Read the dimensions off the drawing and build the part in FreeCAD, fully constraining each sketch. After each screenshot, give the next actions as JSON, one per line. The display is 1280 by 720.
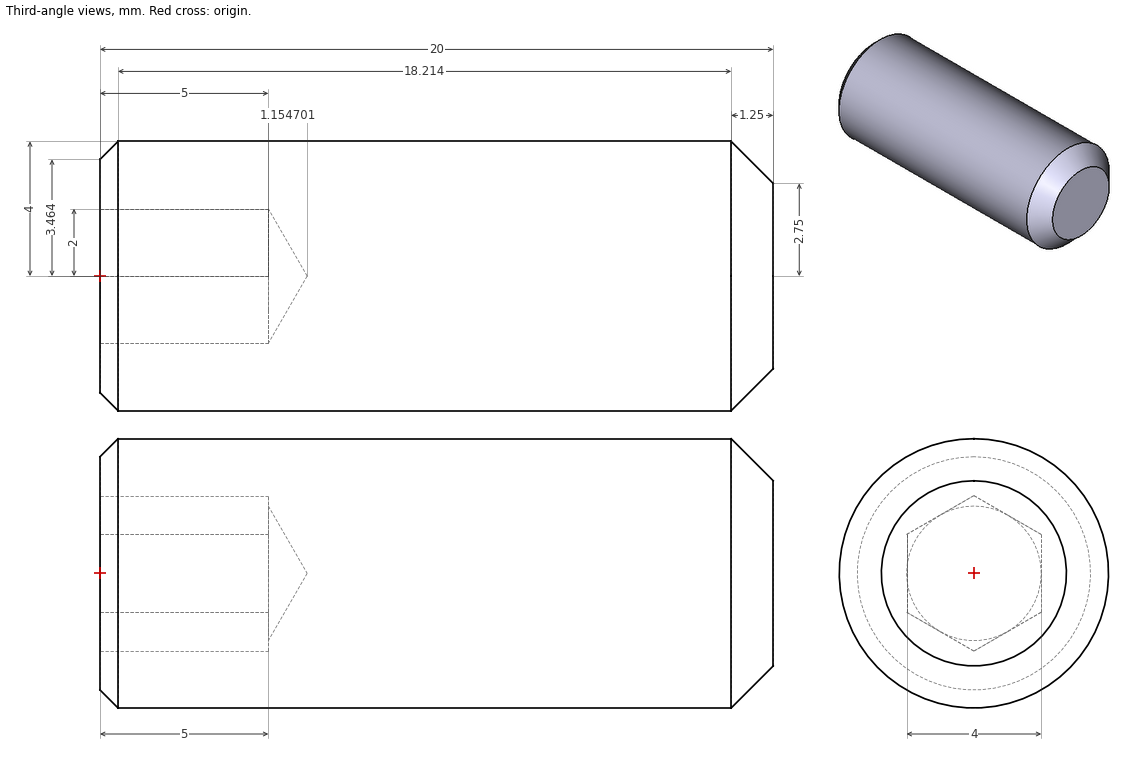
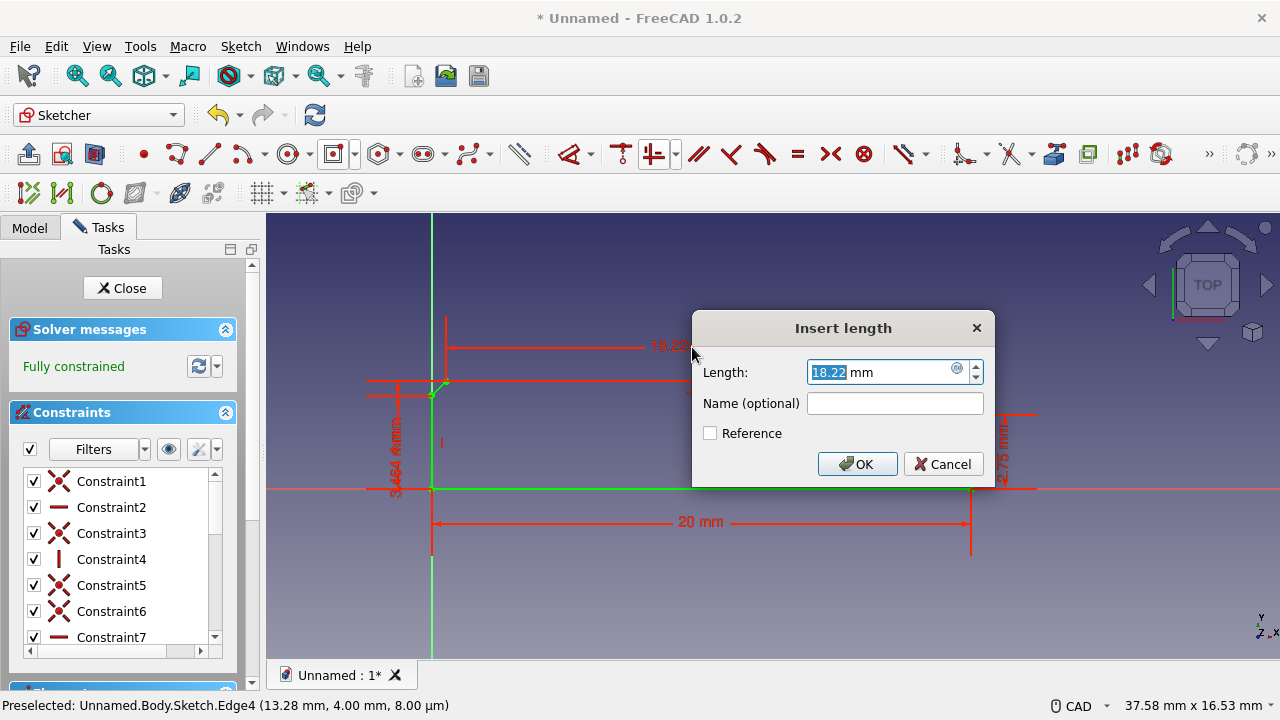
{"action": "type", "text": "18.214"}
{"action": "key", "text": "Return"}
{"action": "key", "text": "Escape"}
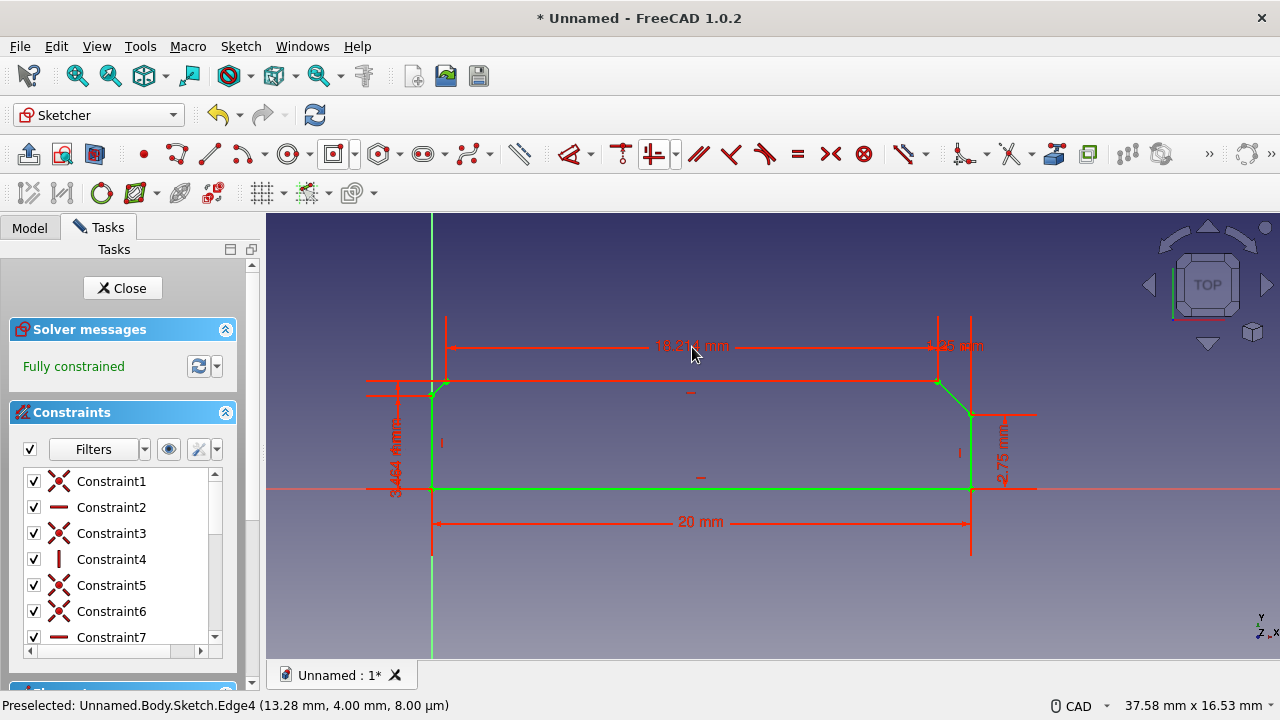
{"action": "left_click", "coordinate": [123, 288]}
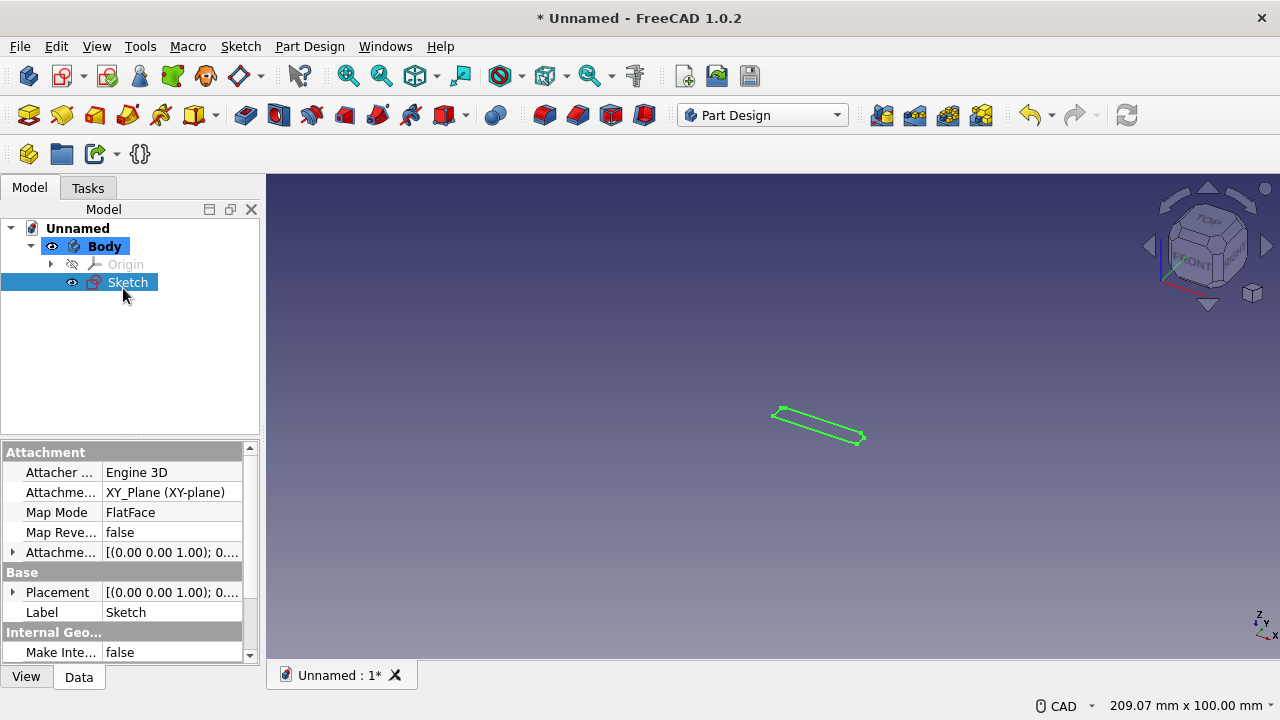
{"action": "left_click", "coordinate": [62, 116]}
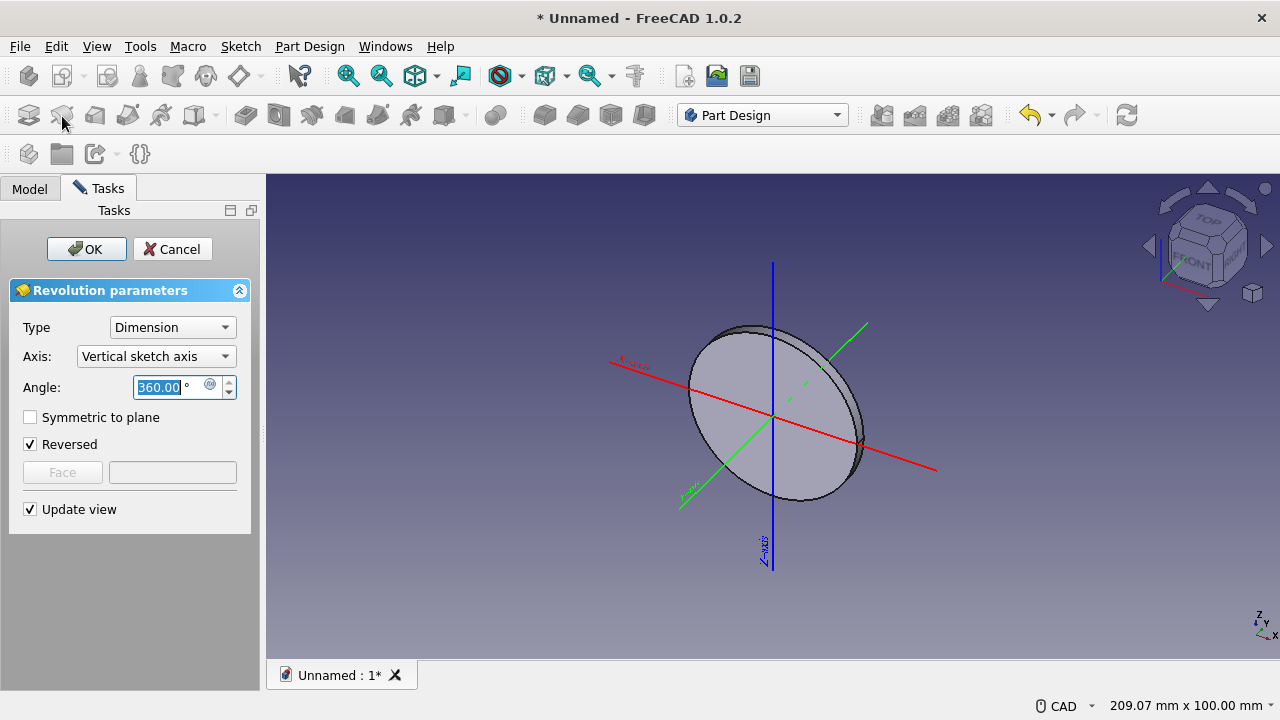
{"action": "left_click", "coordinate": [157, 356]}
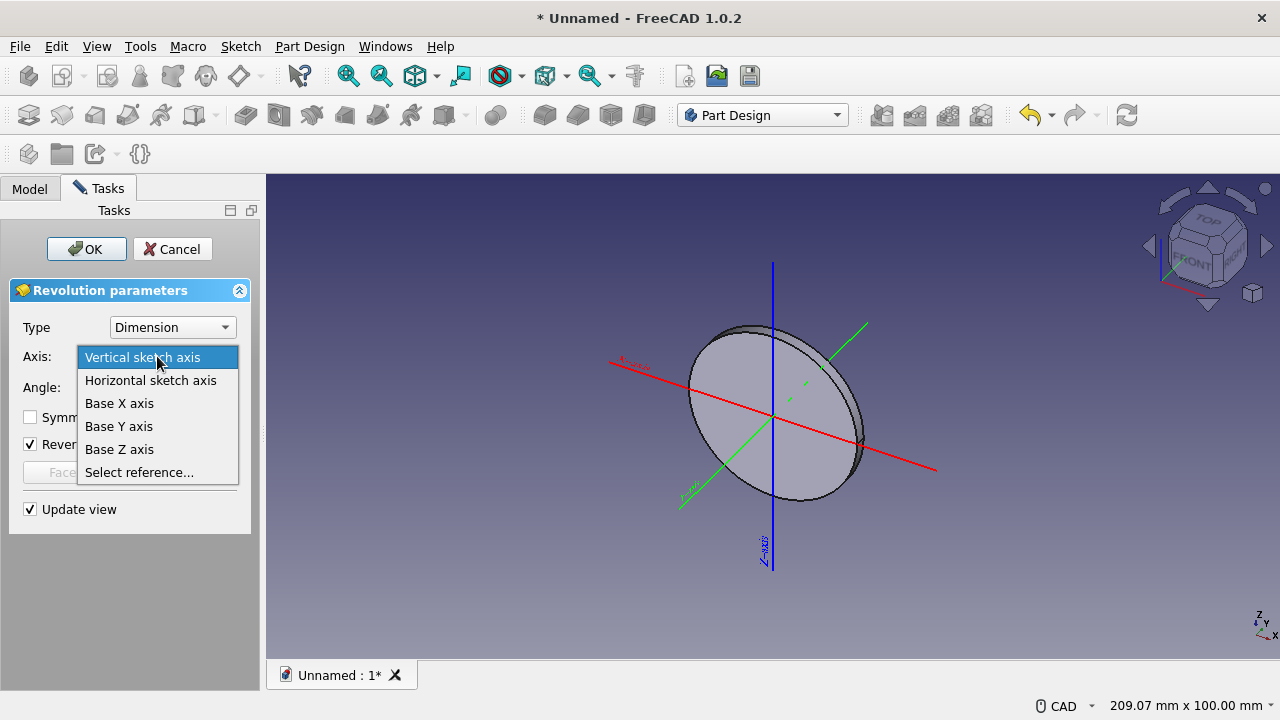
{"action": "left_click", "coordinate": [156, 380]}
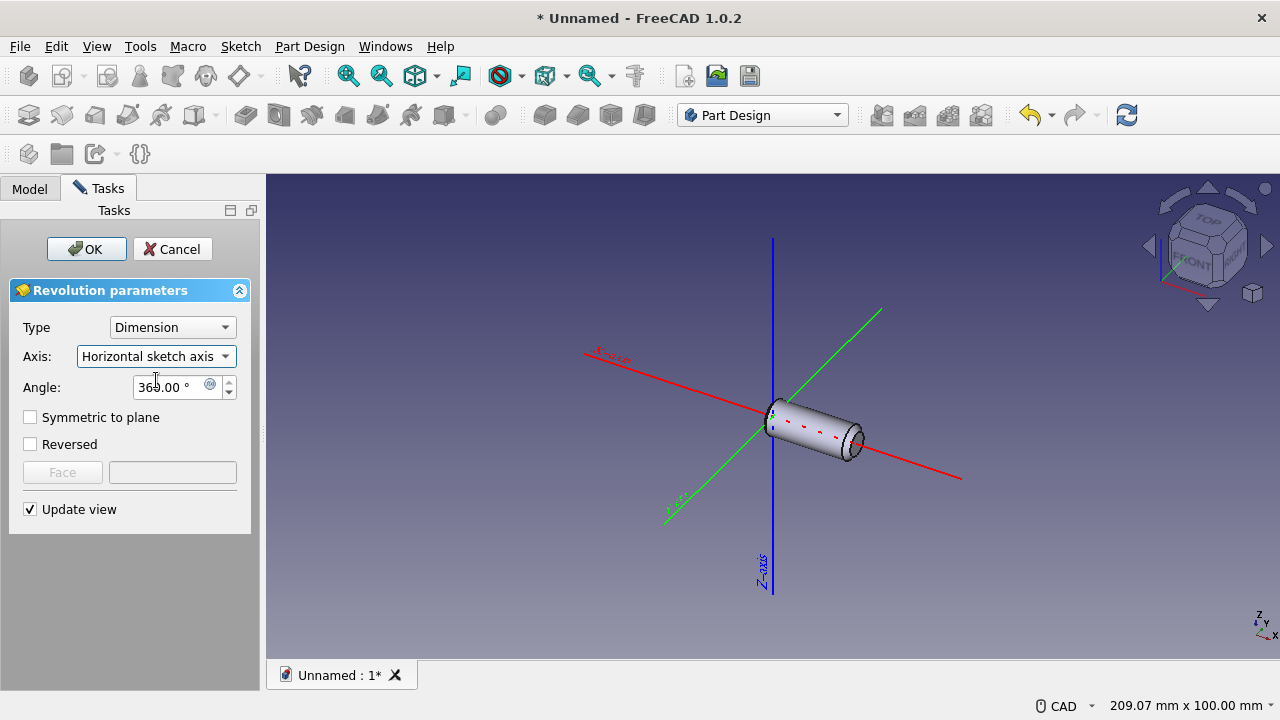
{"action": "left_click", "coordinate": [87, 249]}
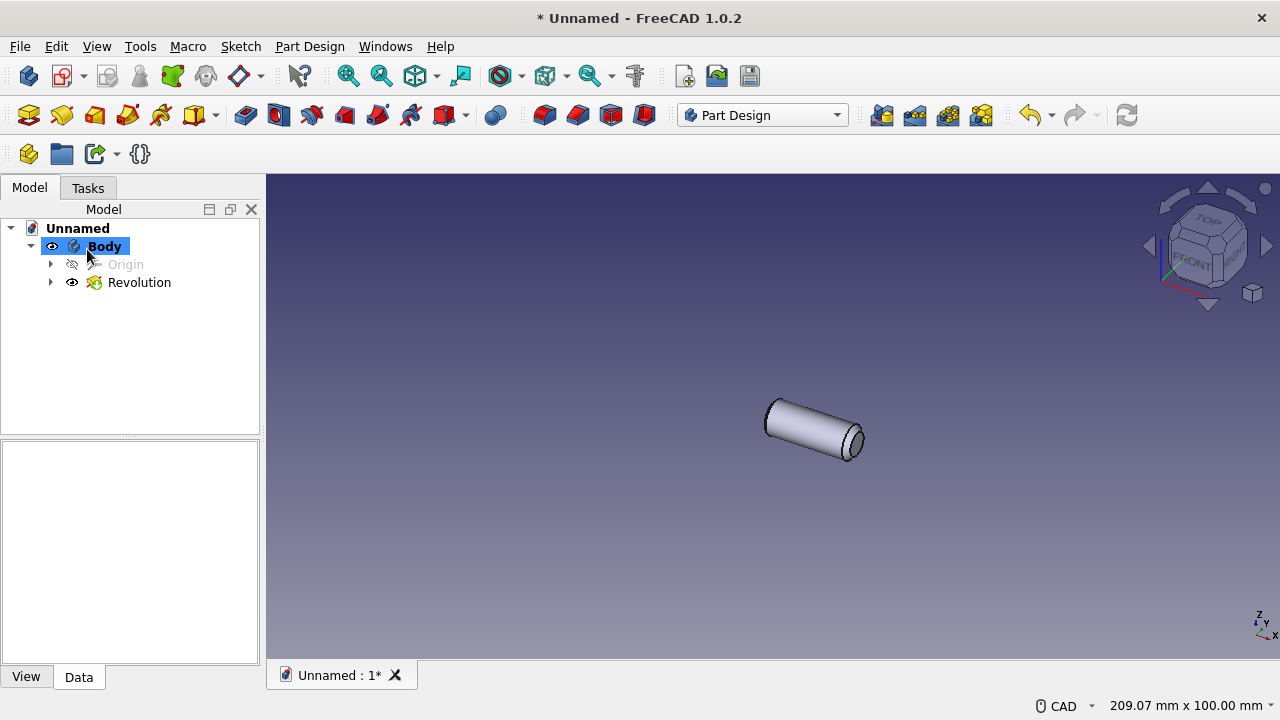
{"action": "left_click", "coordinate": [349, 76]}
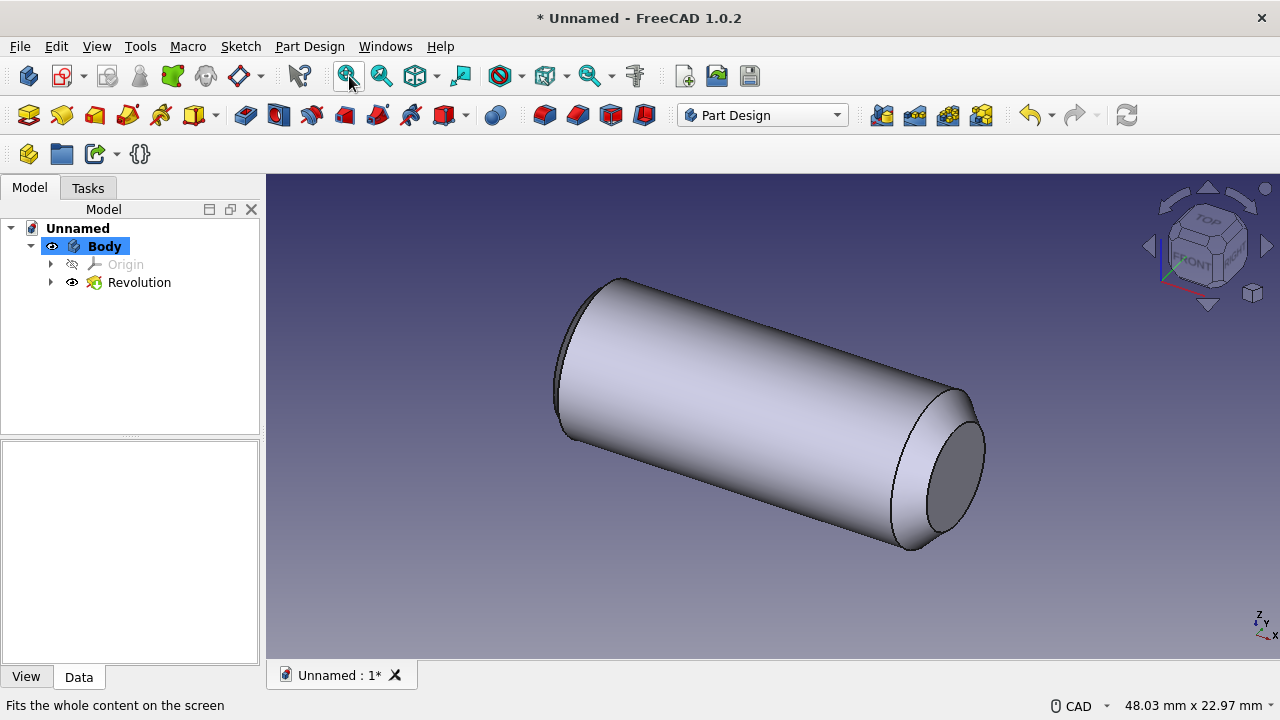
{"action": "left_click", "coordinate": [62, 76]}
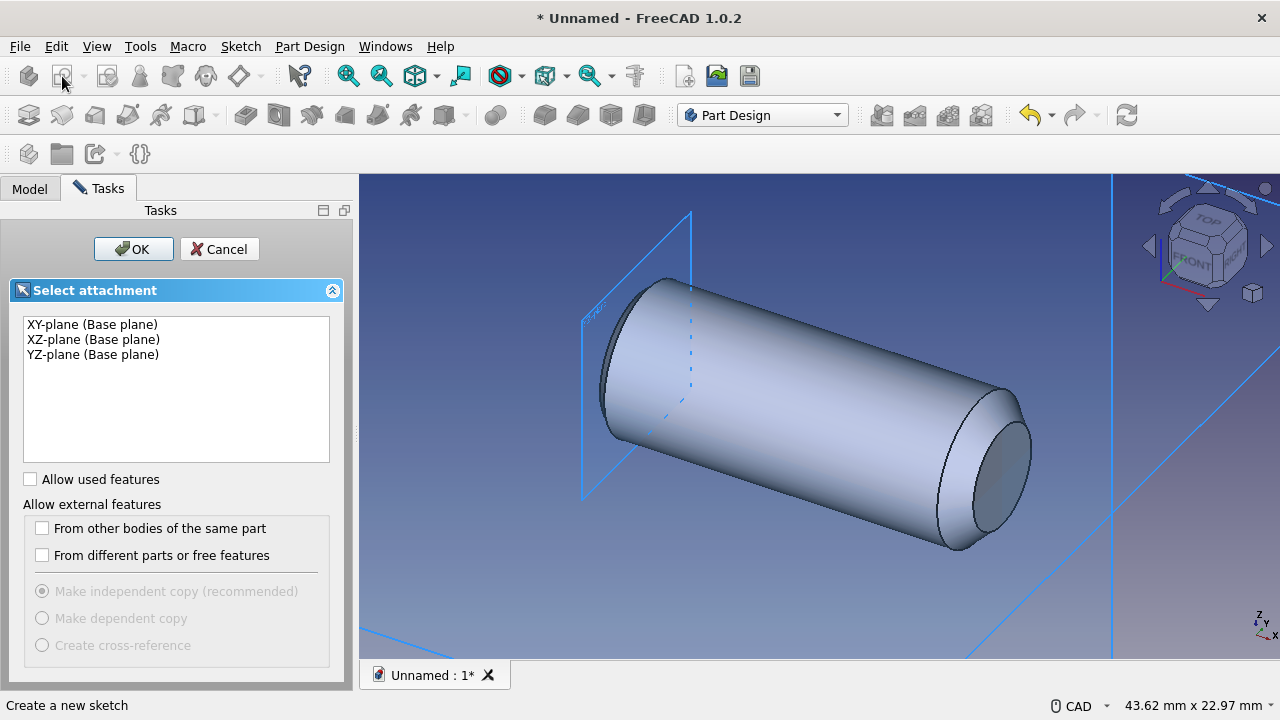
{"action": "left_click", "coordinate": [84, 354]}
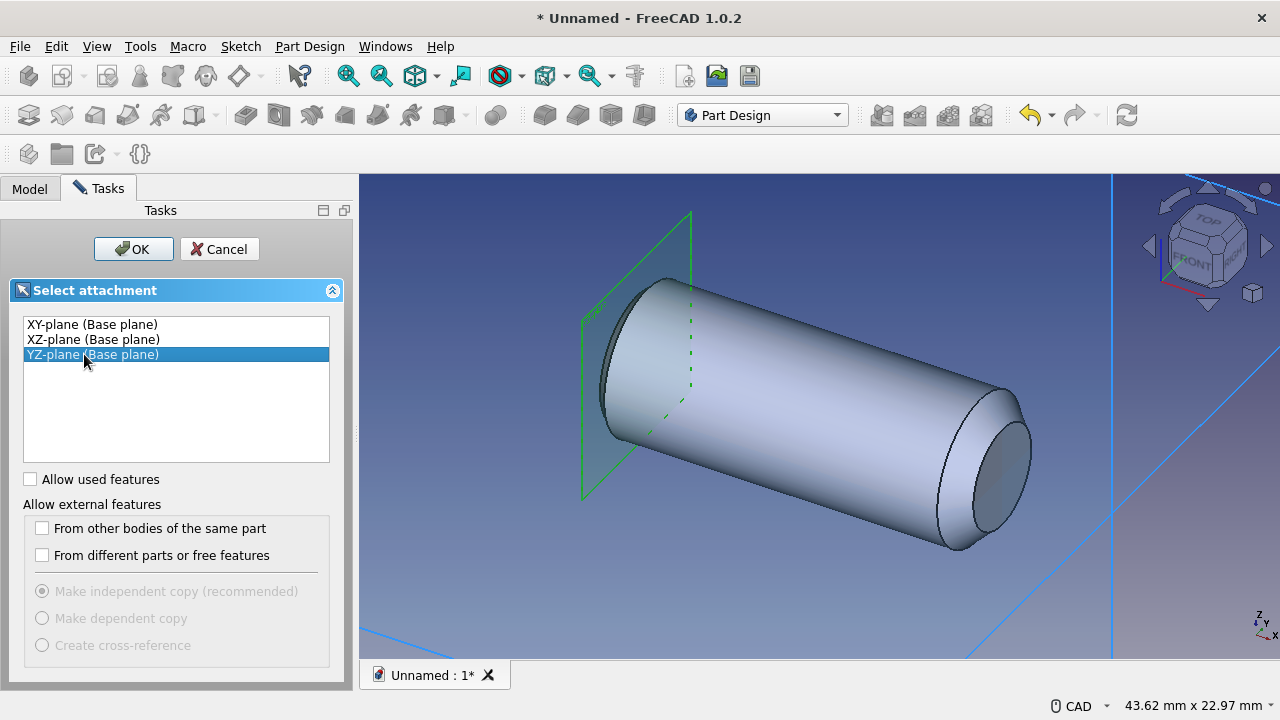
{"action": "left_click", "coordinate": [134, 249]}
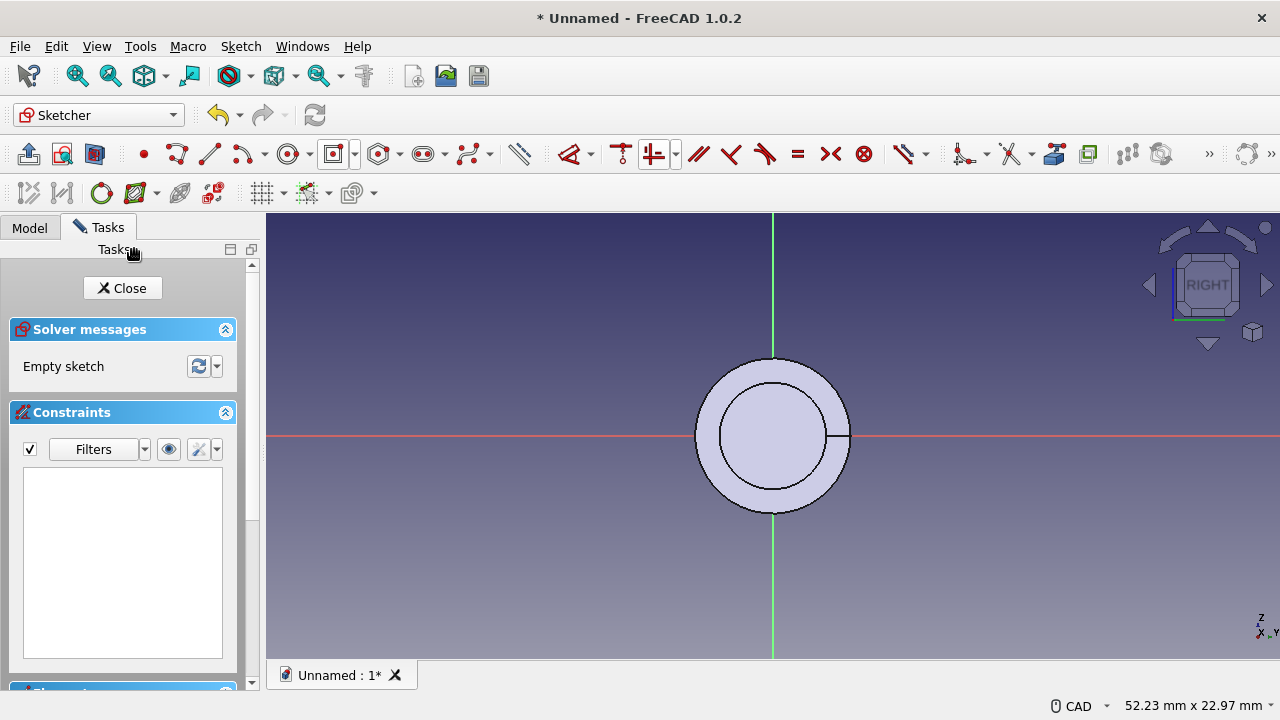
{"action": "left_click", "coordinate": [95, 154]}